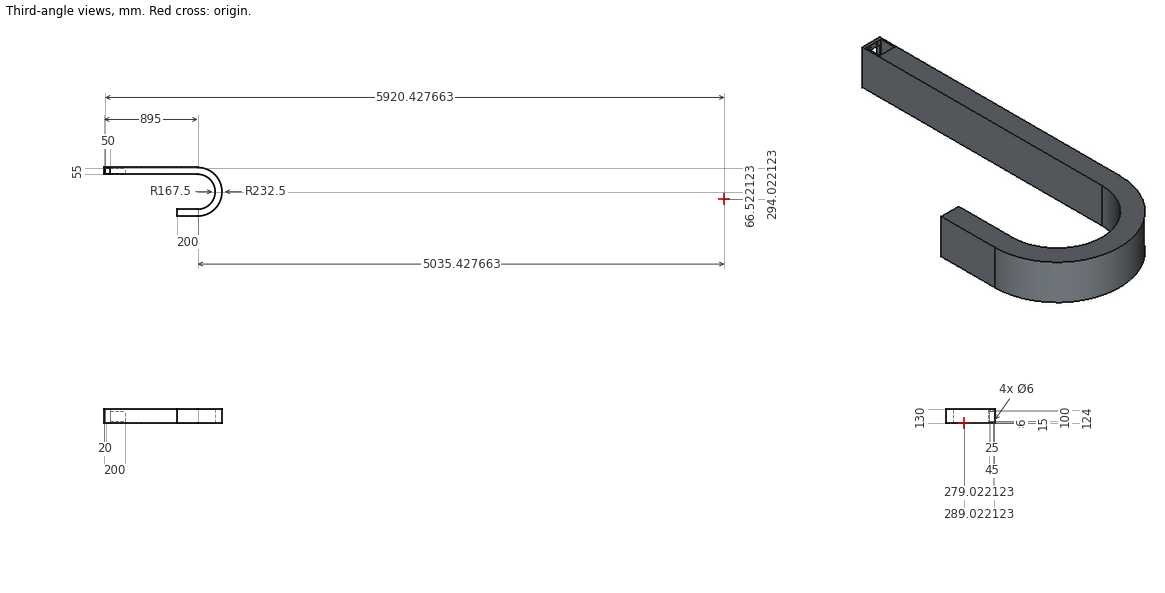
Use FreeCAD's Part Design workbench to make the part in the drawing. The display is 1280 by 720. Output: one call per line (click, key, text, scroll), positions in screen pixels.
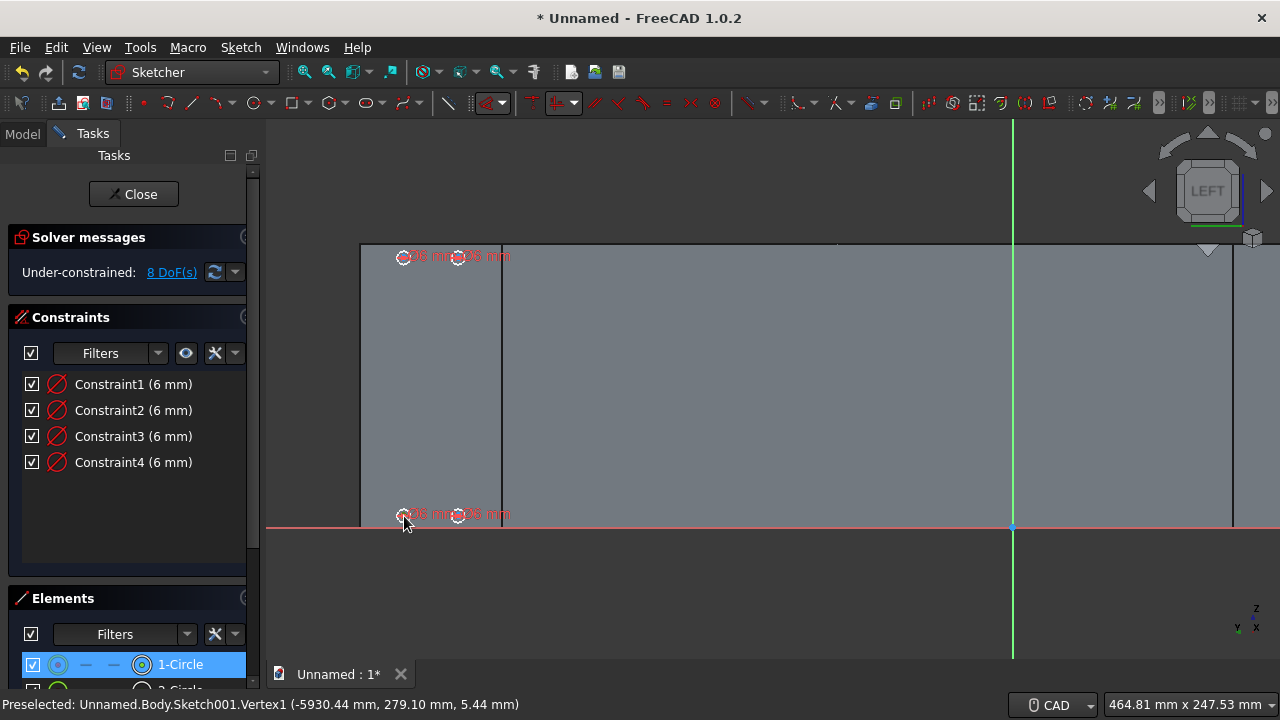
click(458, 516)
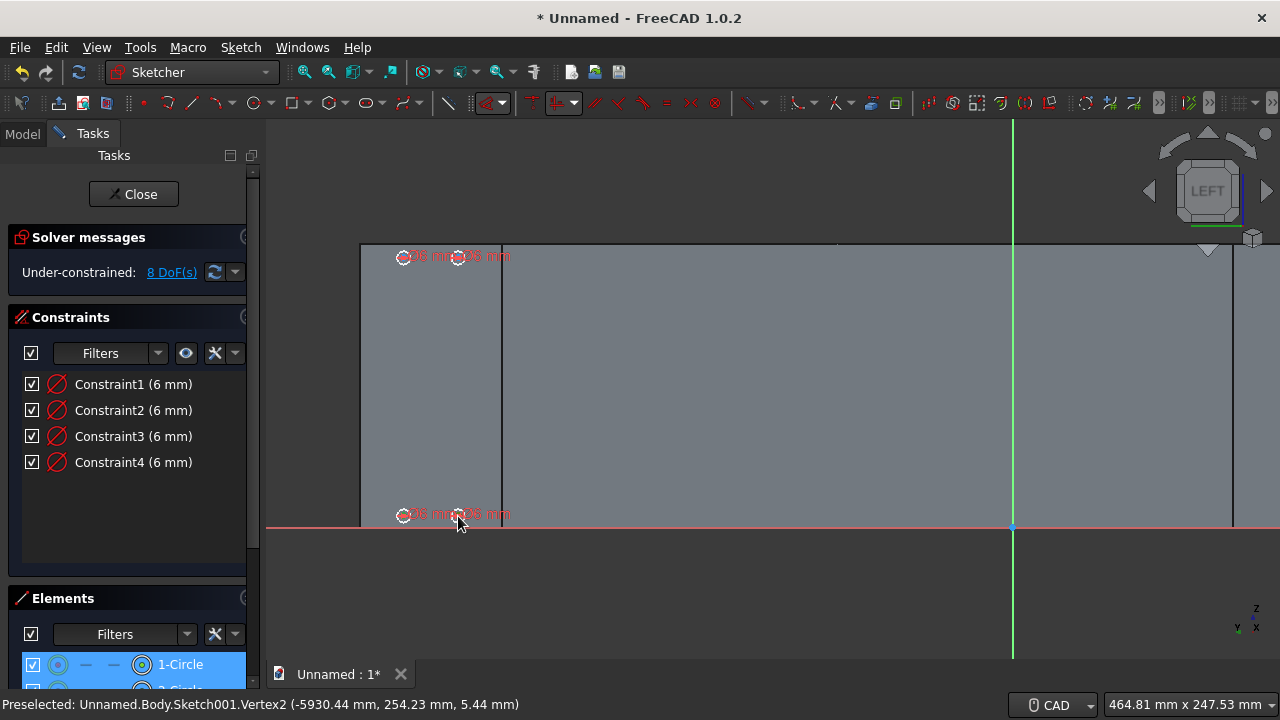
click(576, 104)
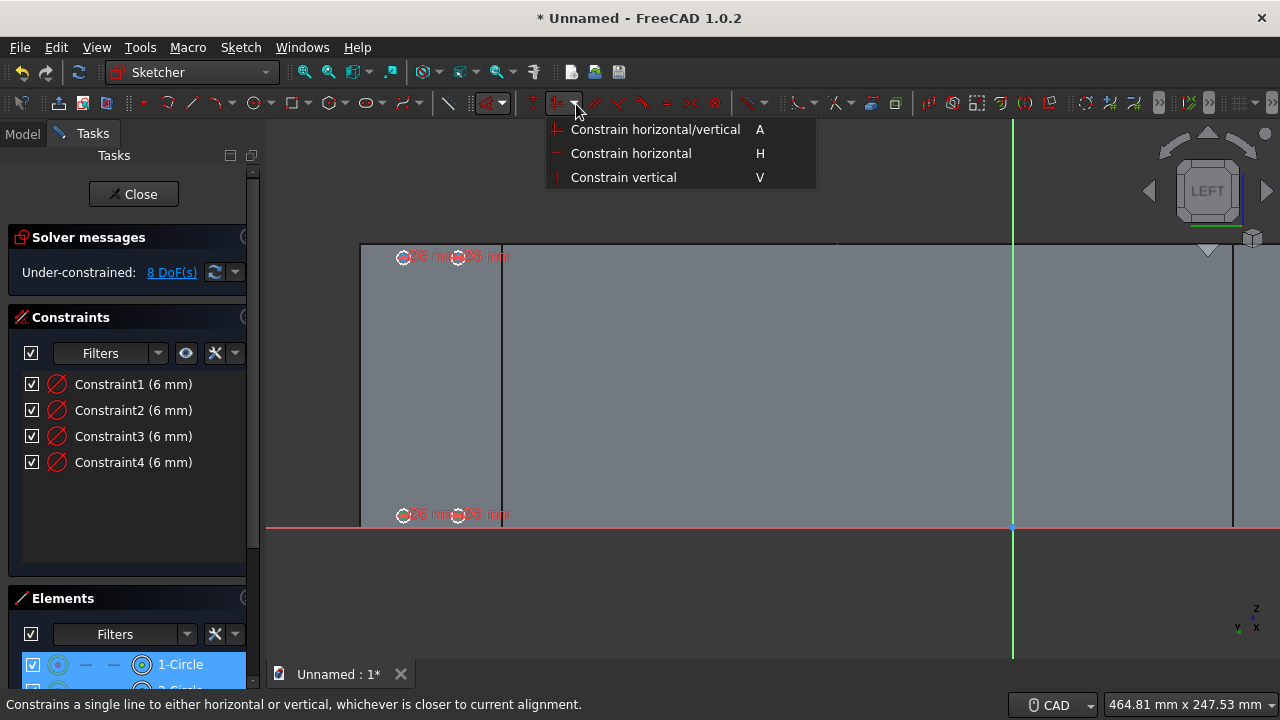
click(681, 153)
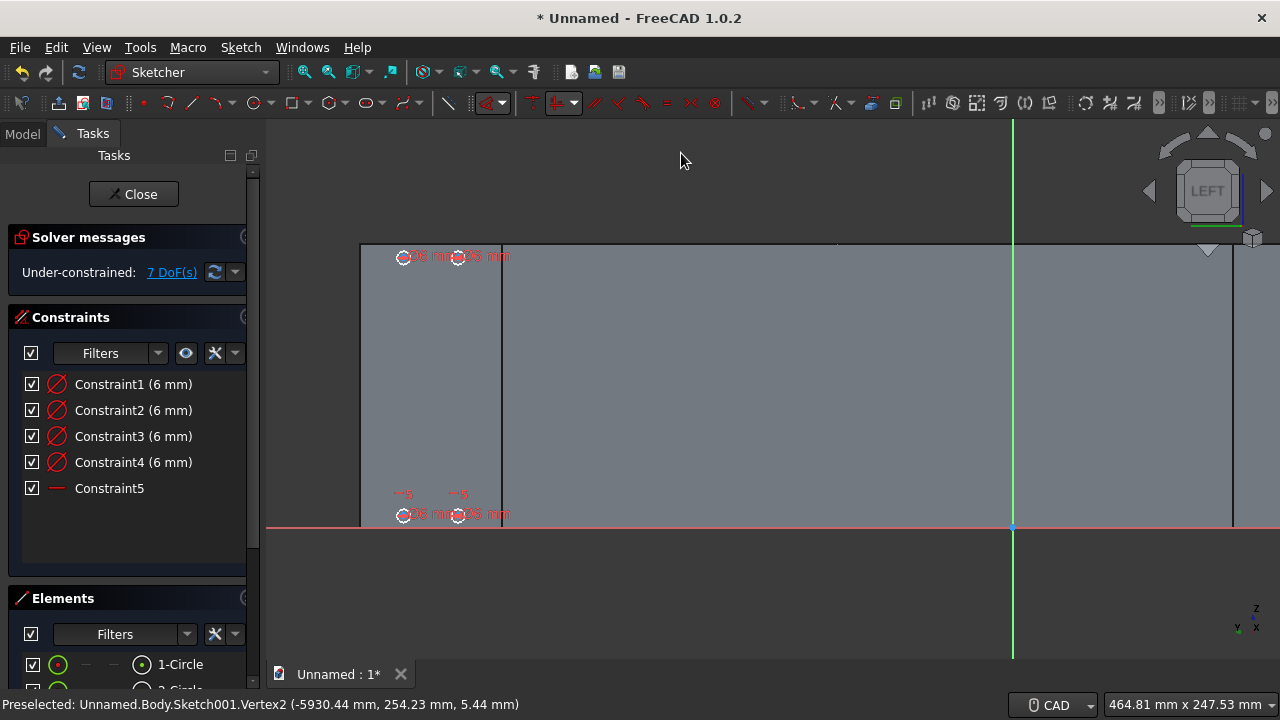
click(404, 516)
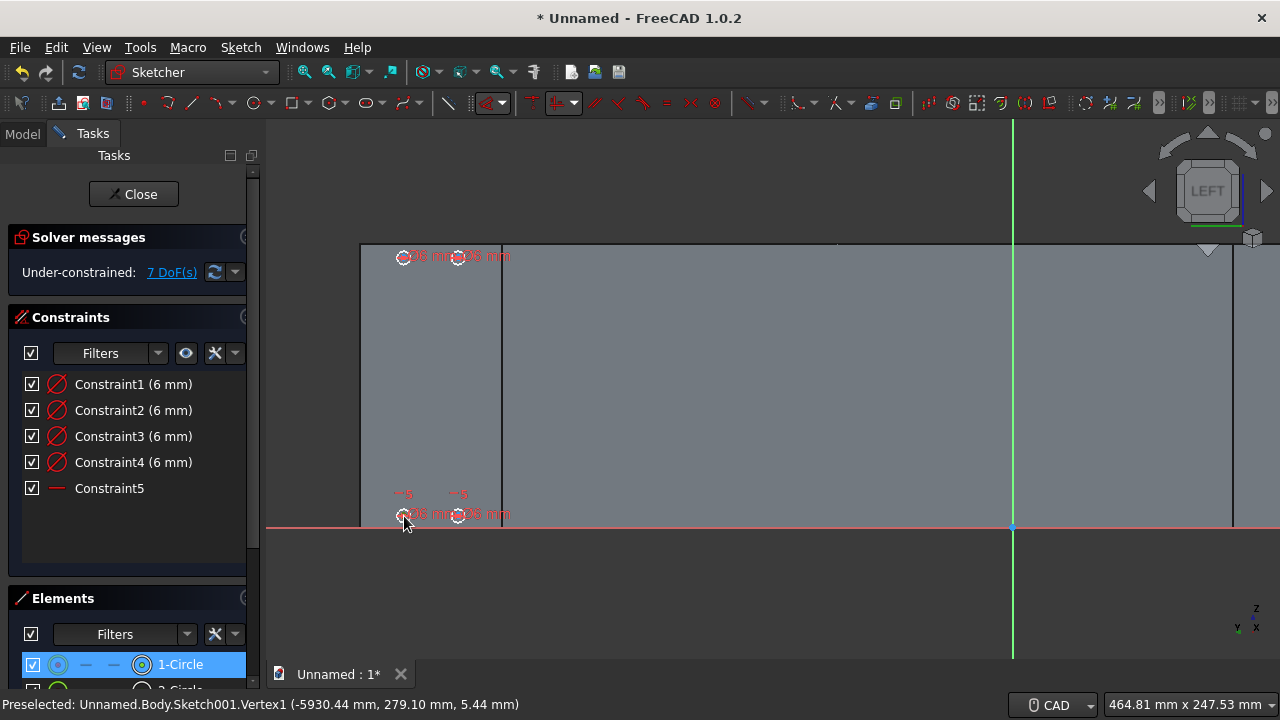
click(404, 258)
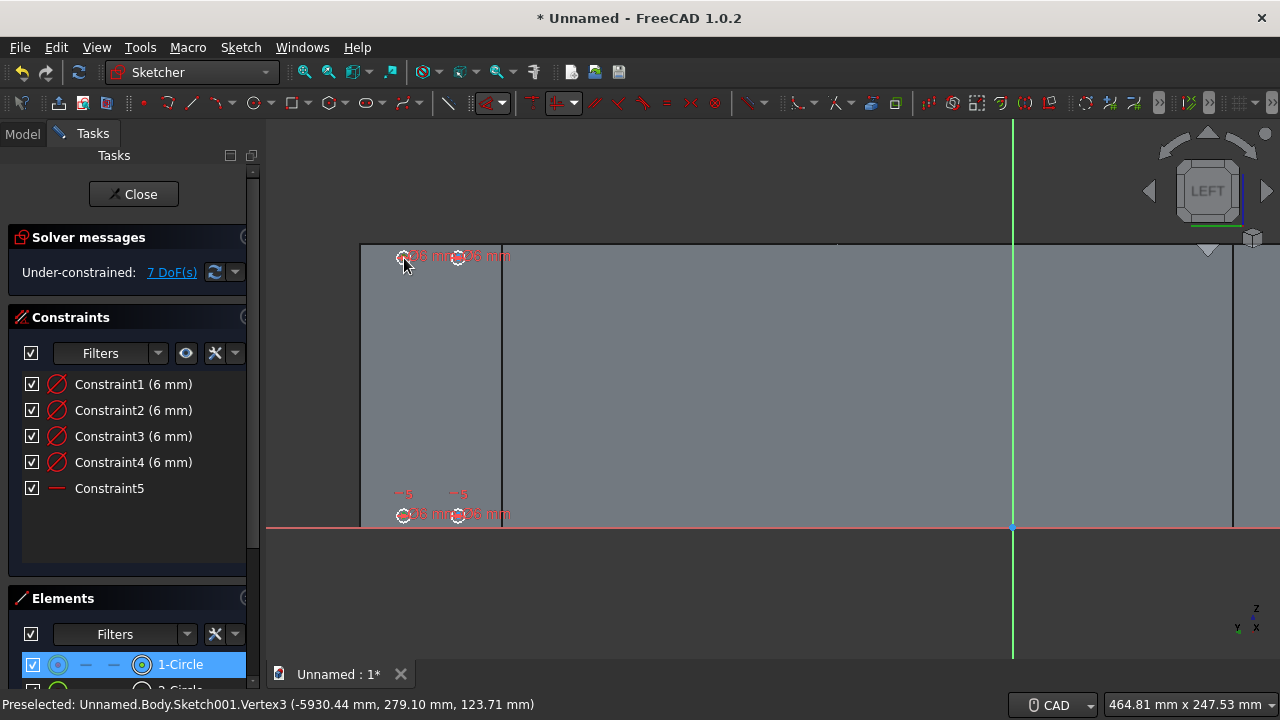
key(v)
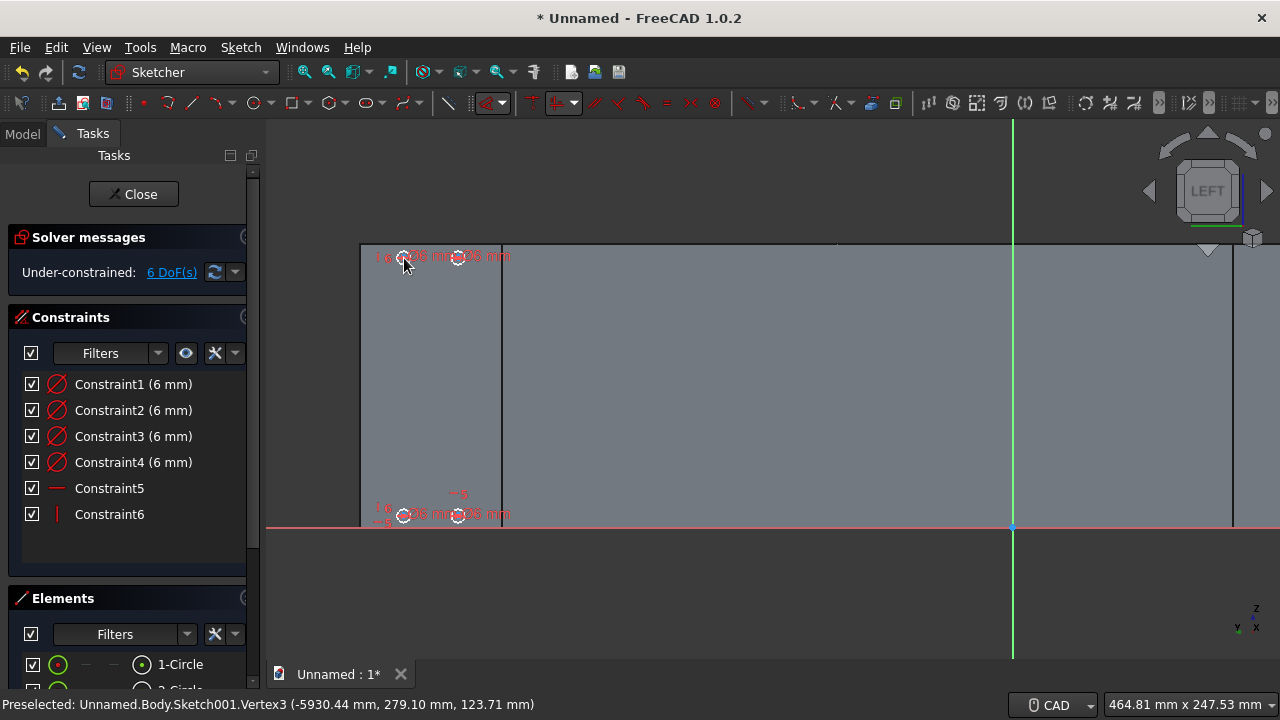
click(458, 516)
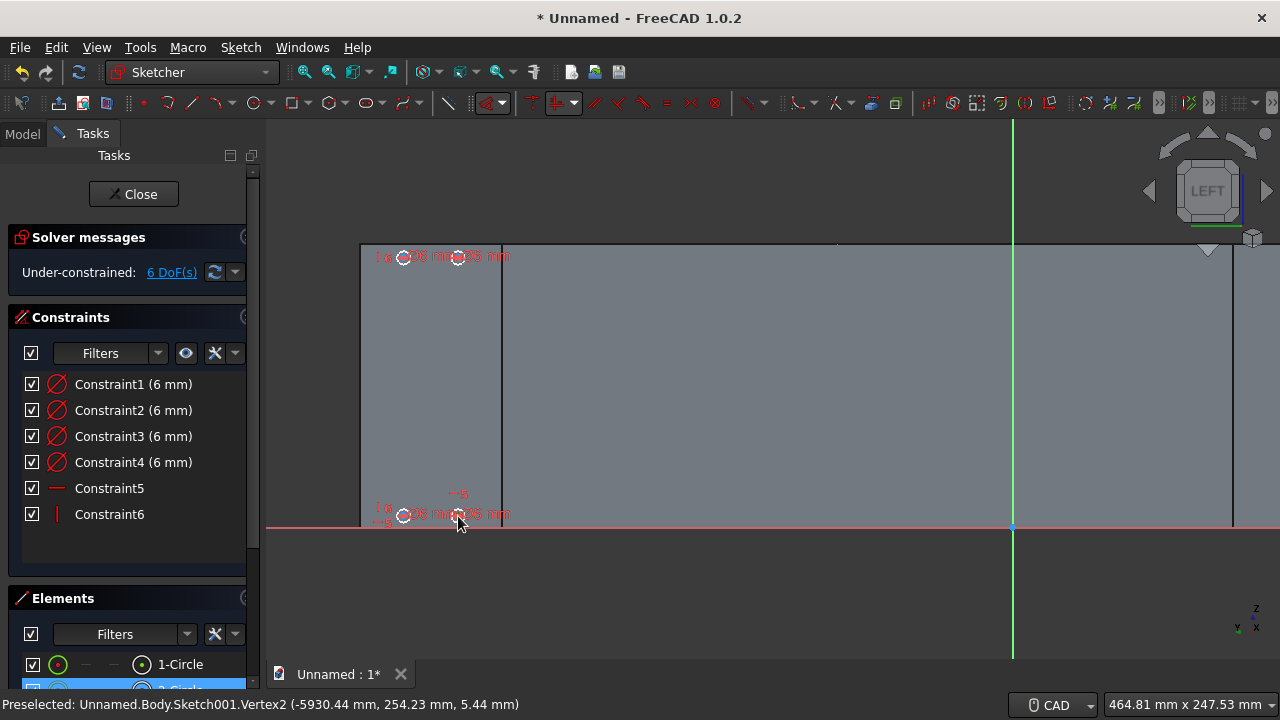
click(458, 258)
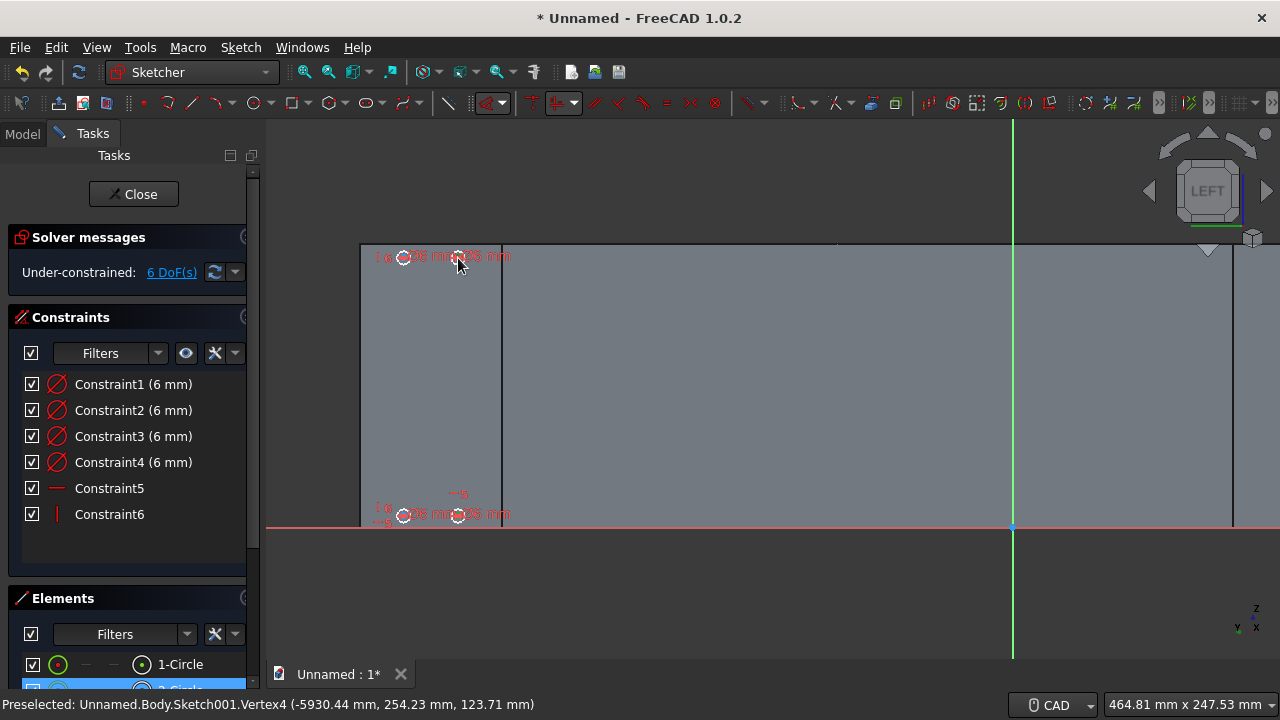
key(v)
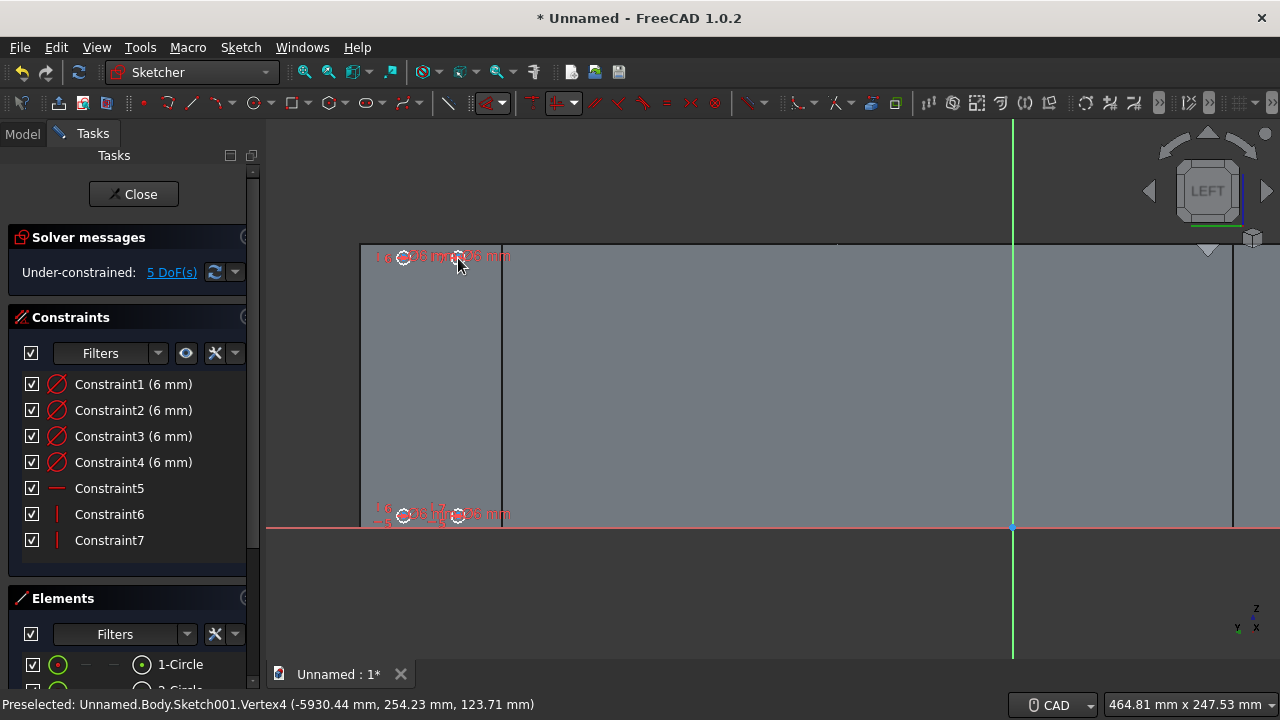
click(404, 258)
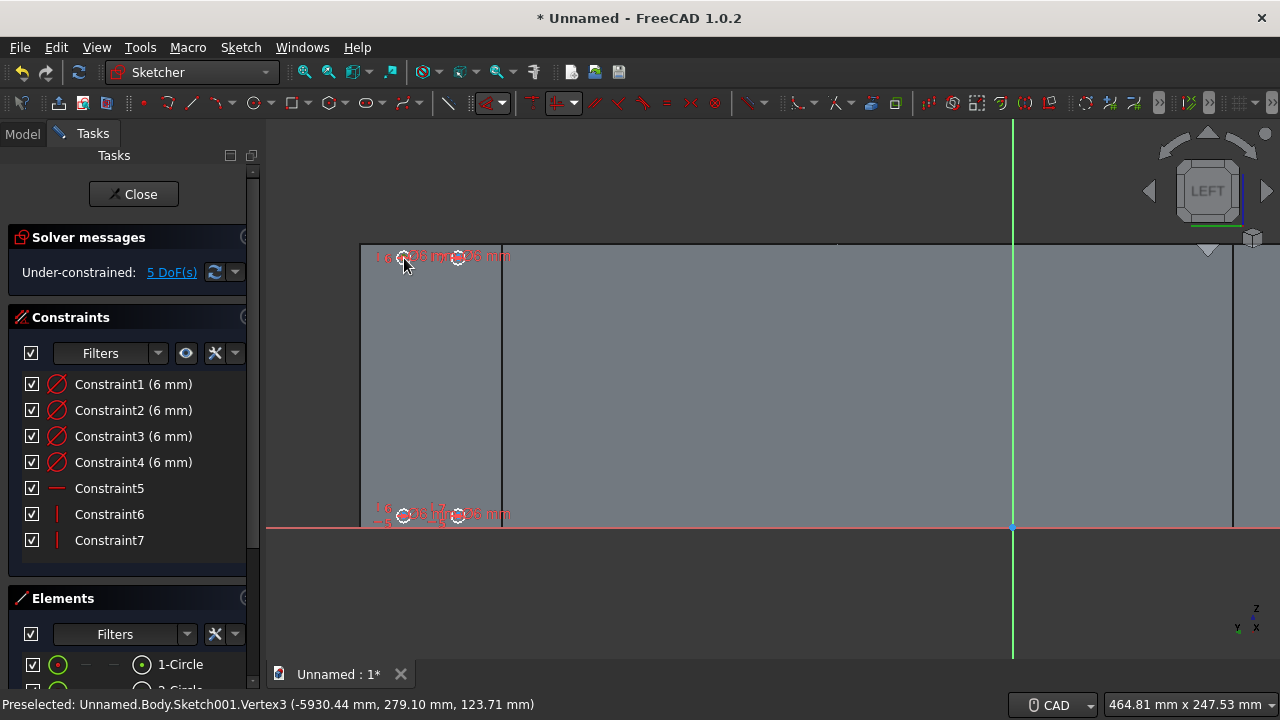
click(458, 258)